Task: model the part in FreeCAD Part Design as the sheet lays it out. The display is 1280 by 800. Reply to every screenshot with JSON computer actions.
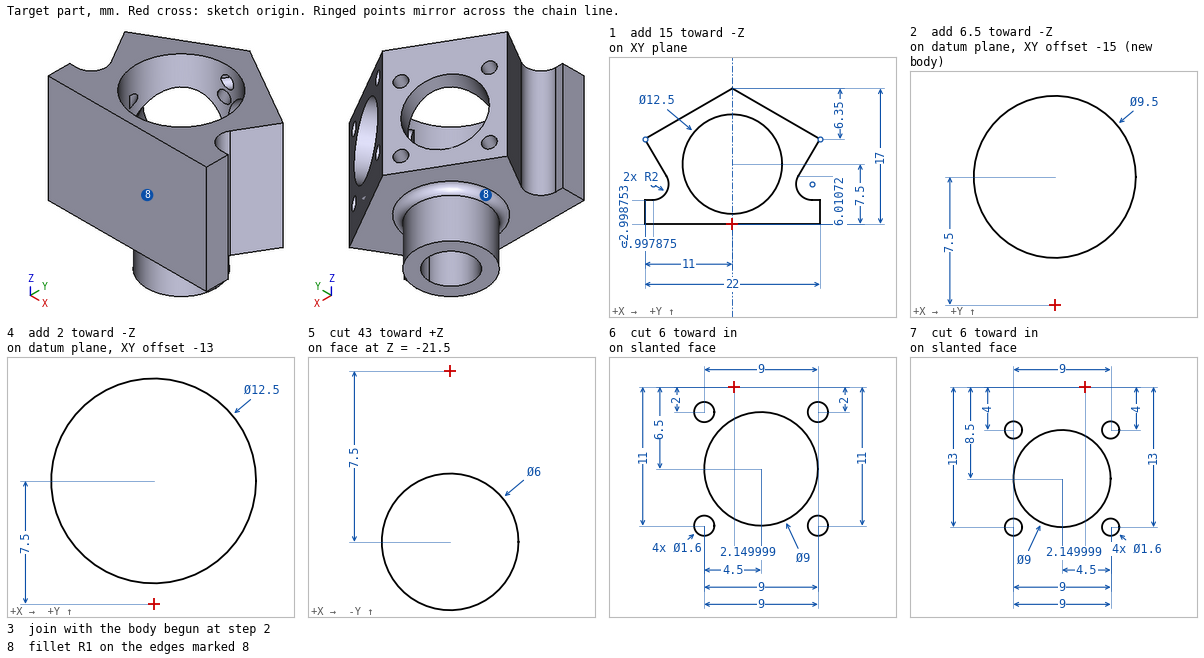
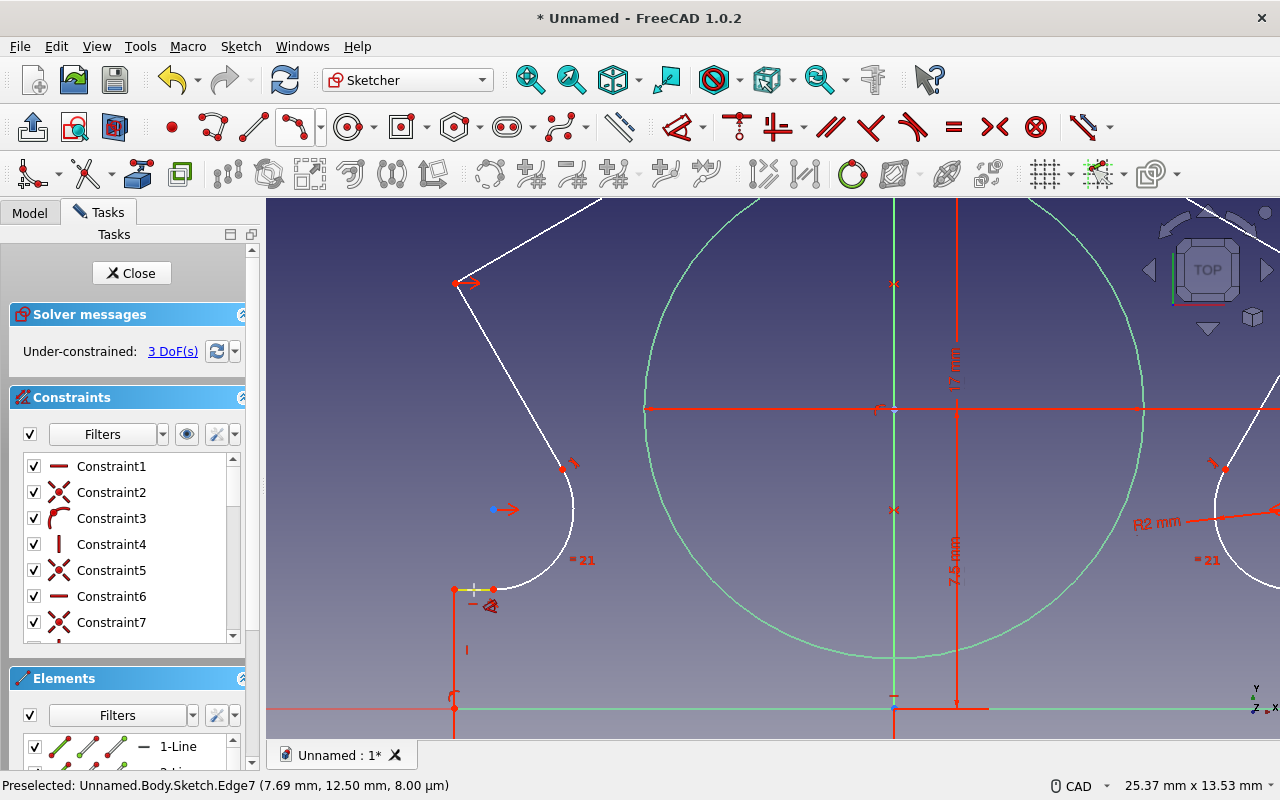
{"action": "left_click", "coordinate": [474, 590]}
{"action": "left_click", "coordinate": [474, 624]}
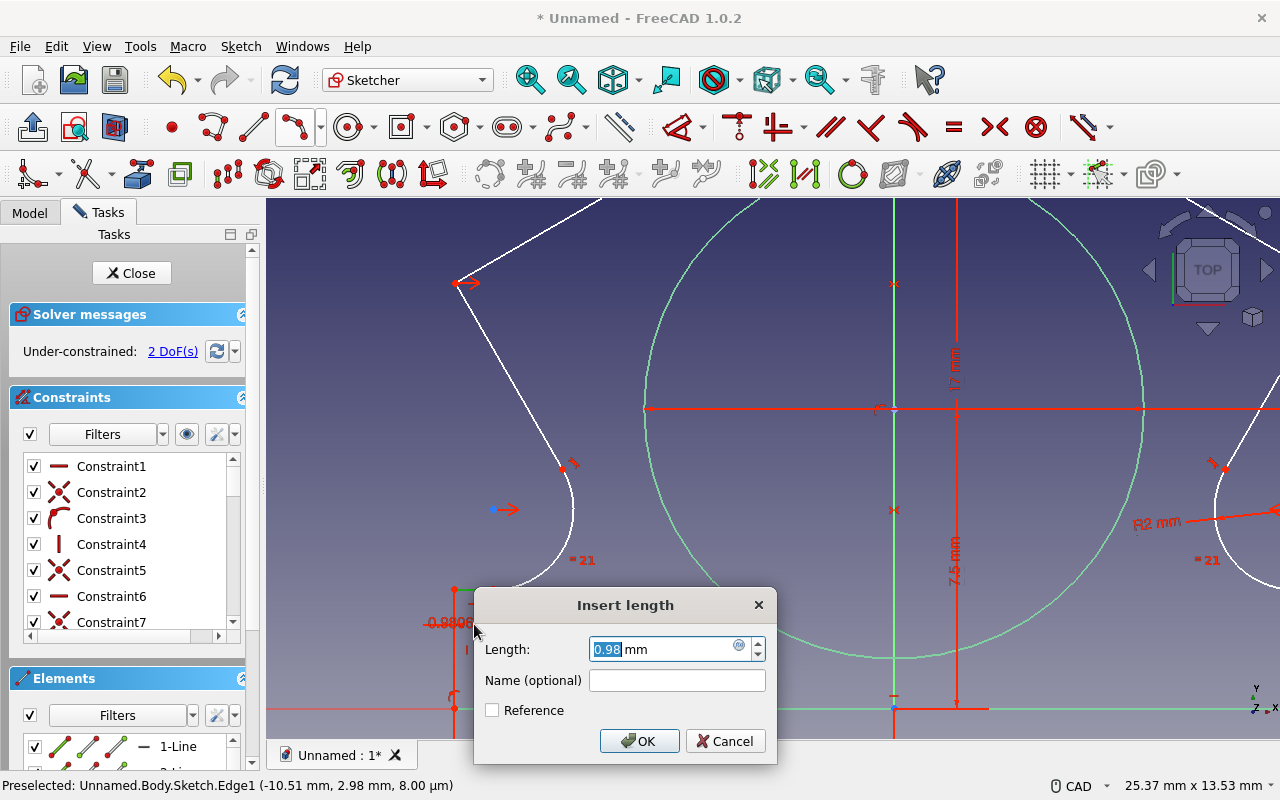
{"action": "type", "text": "0.997875"}
{"action": "key", "text": "Return"}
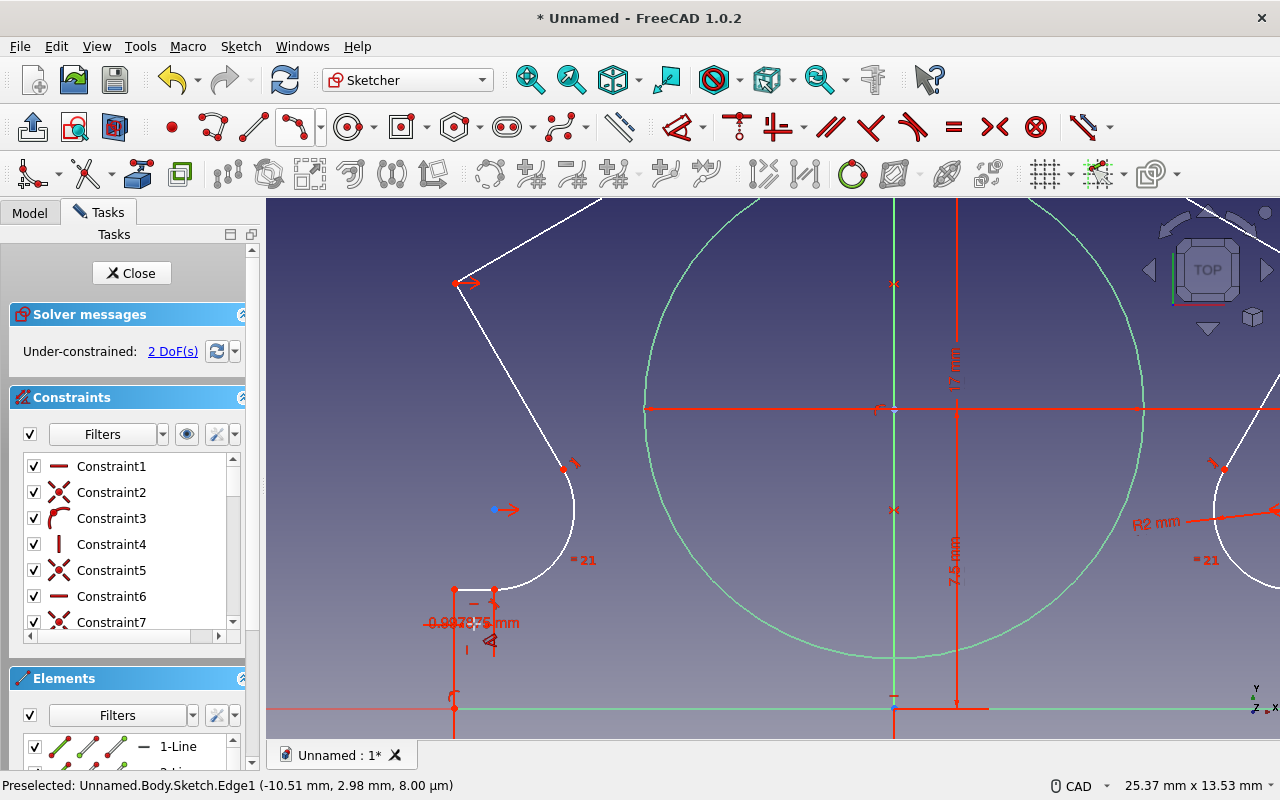
{"action": "left_click", "coordinate": [454, 625]}
{"action": "left_click", "coordinate": [420, 649]}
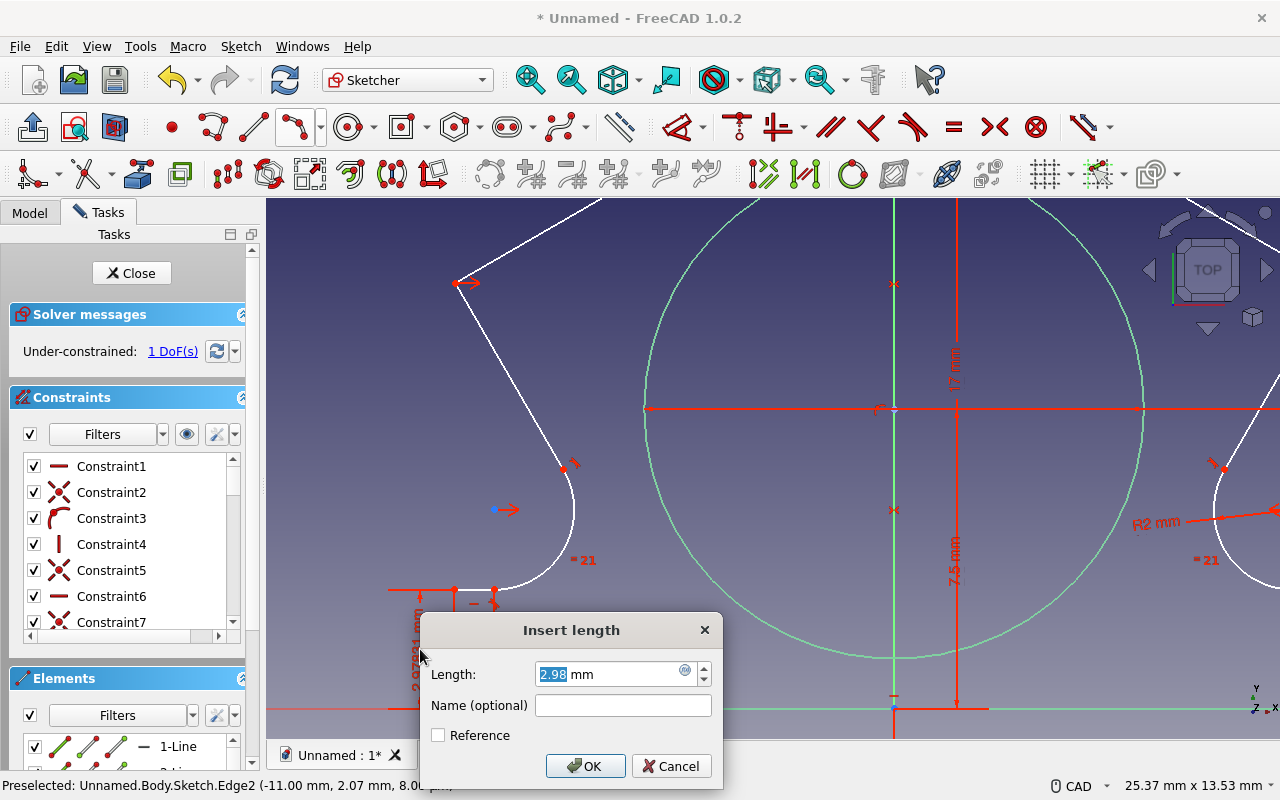
{"action": "type", "text": "2.998753"}
{"action": "key", "text": "Return"}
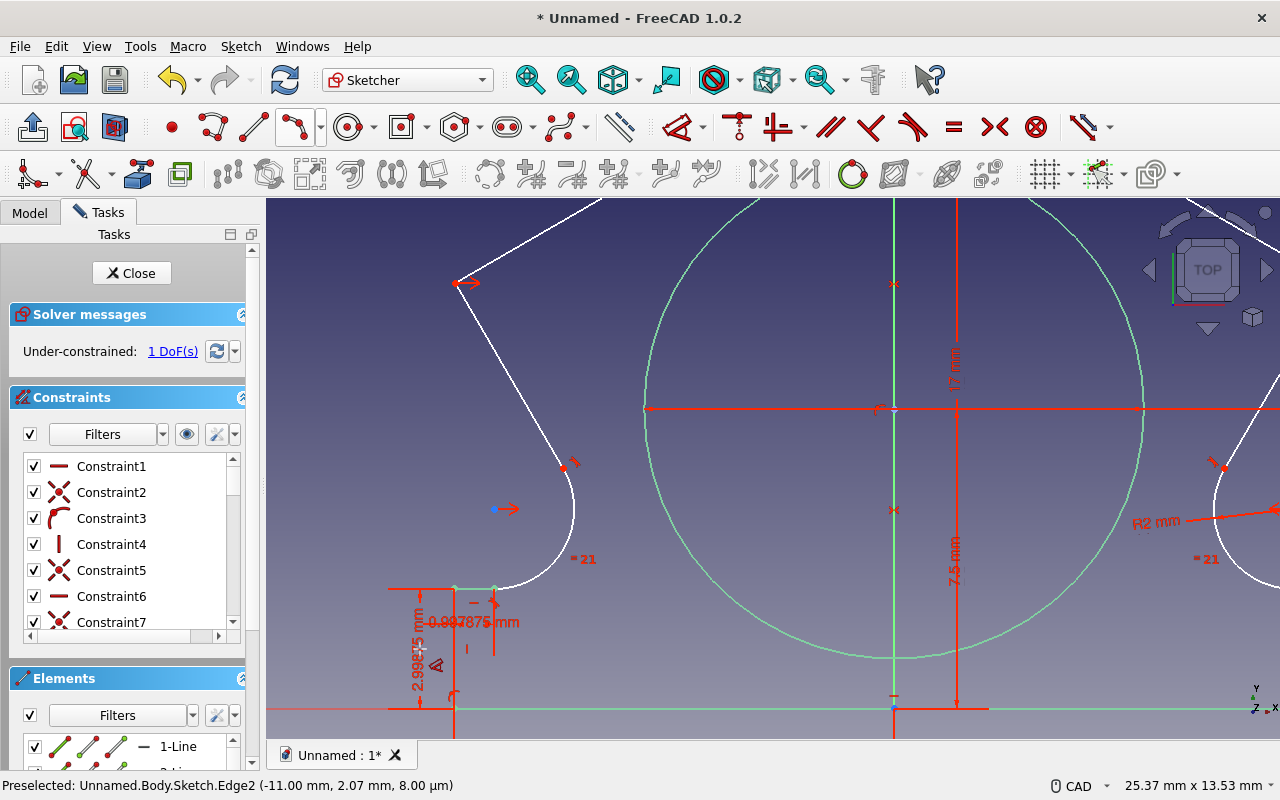
{"action": "scroll", "coordinate": [474, 589], "scroll_direction": "down", "scroll_amount": 3}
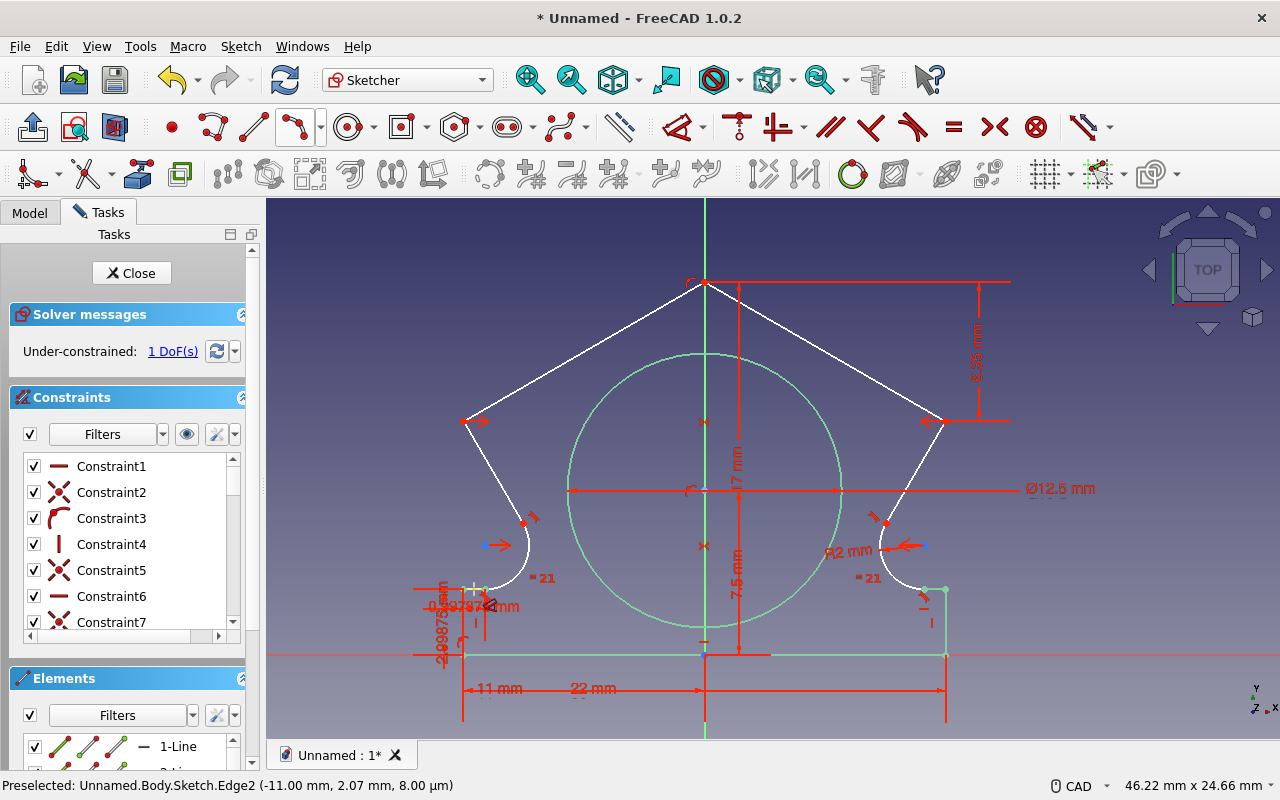
{"action": "left_click", "coordinate": [886, 523]}
{"action": "left_click", "coordinate": [920, 559]}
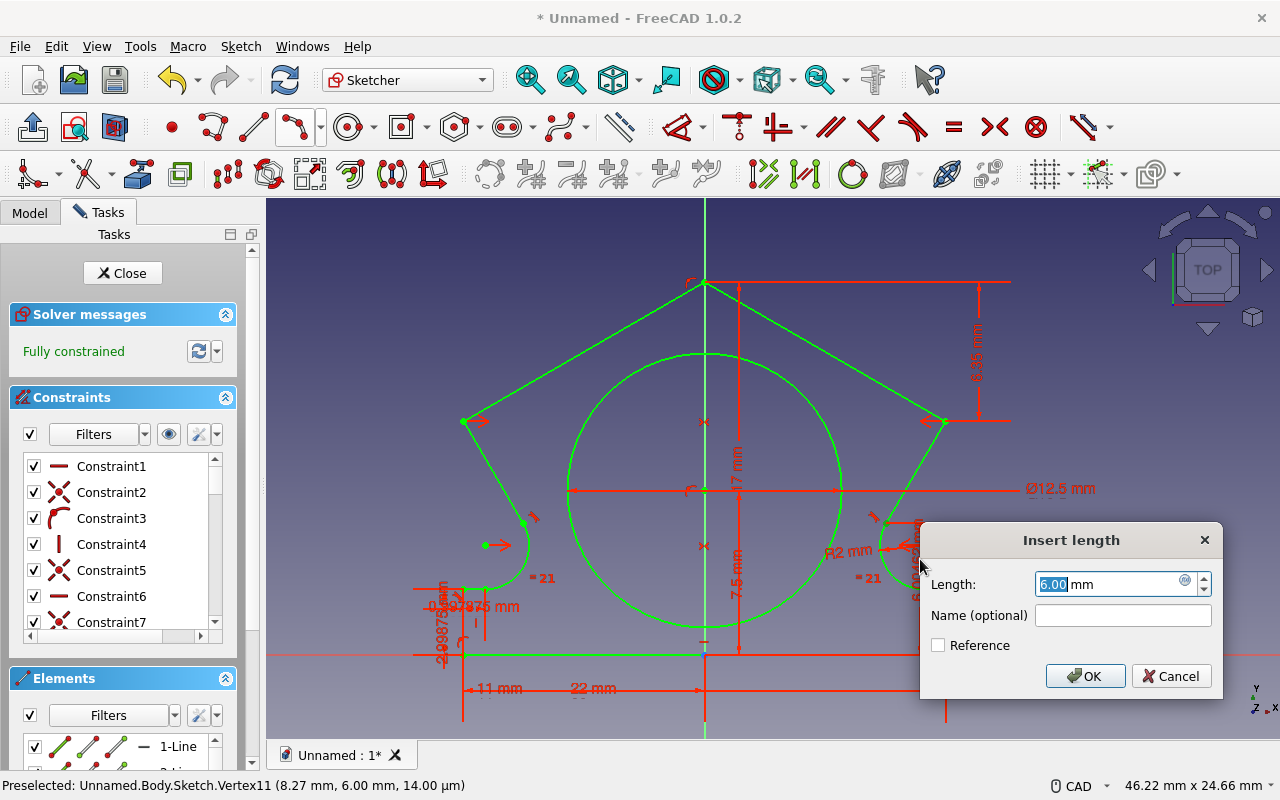
{"action": "type", "text": "6.01072"}
{"action": "key", "text": "Return"}
{"action": "key", "text": "Escape"}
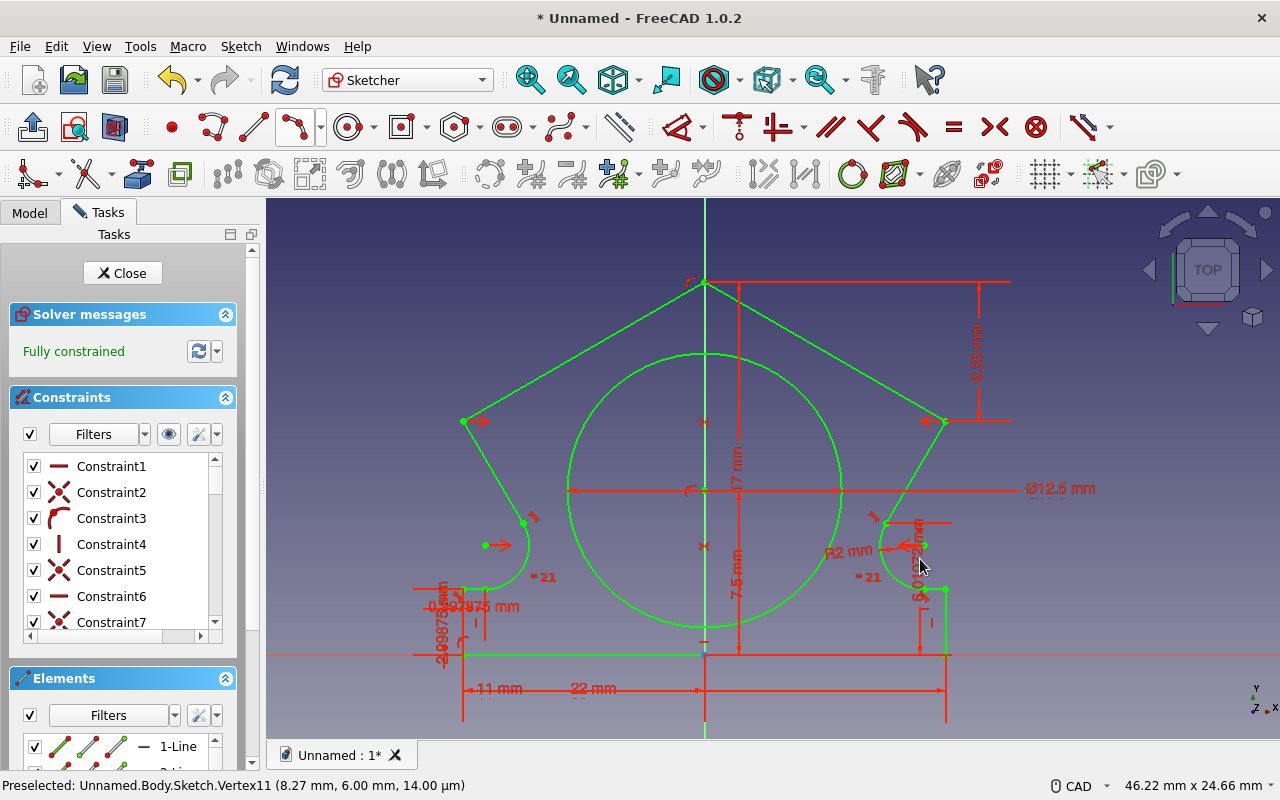
{"action": "left_click", "coordinate": [123, 273]}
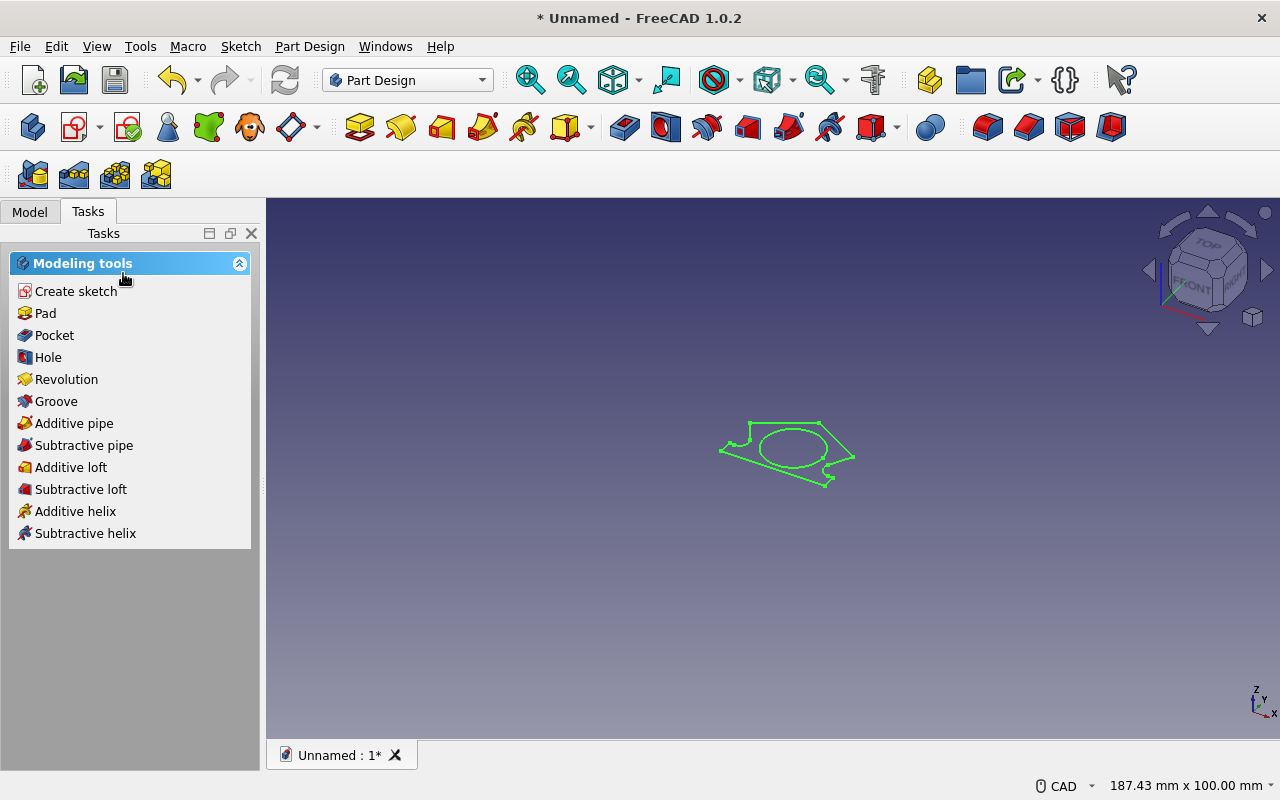
{"action": "left_click", "coordinate": [360, 128]}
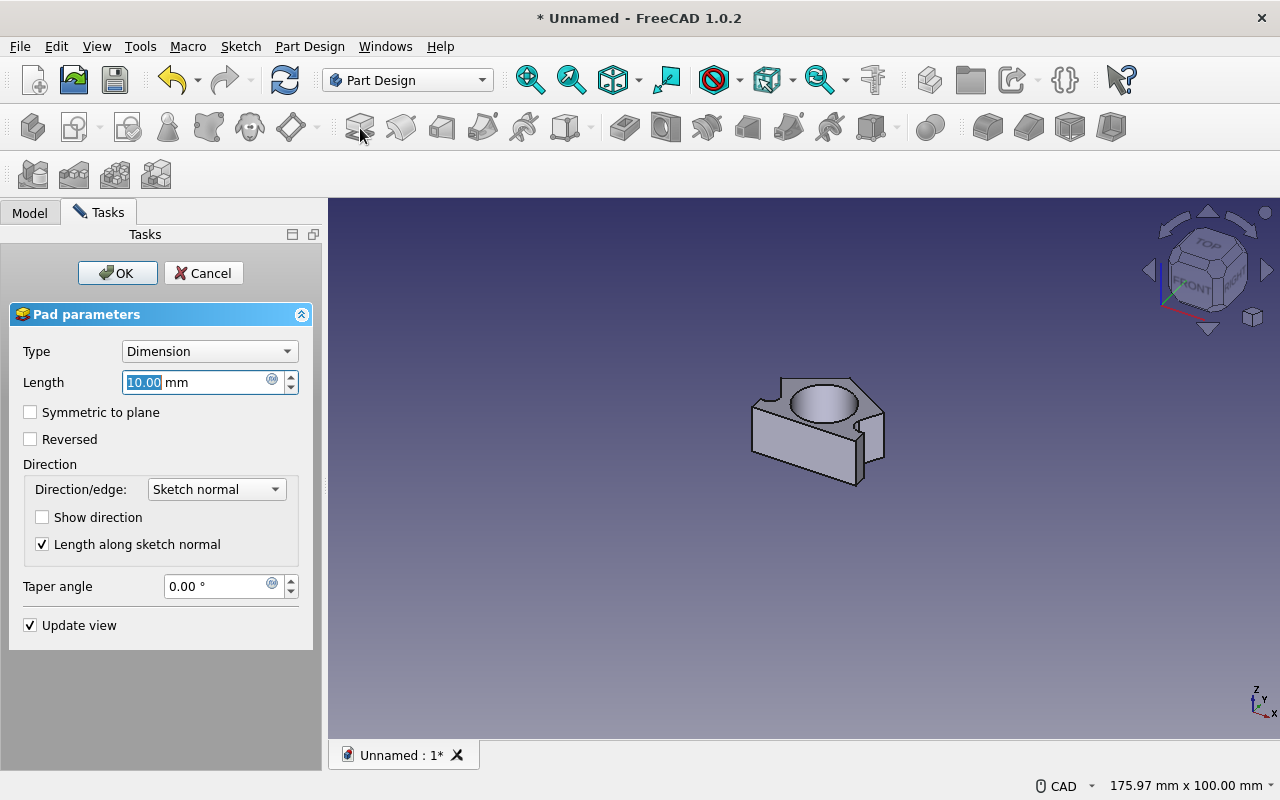
{"action": "type", "text": "15"}
{"action": "key", "text": "Tab"}